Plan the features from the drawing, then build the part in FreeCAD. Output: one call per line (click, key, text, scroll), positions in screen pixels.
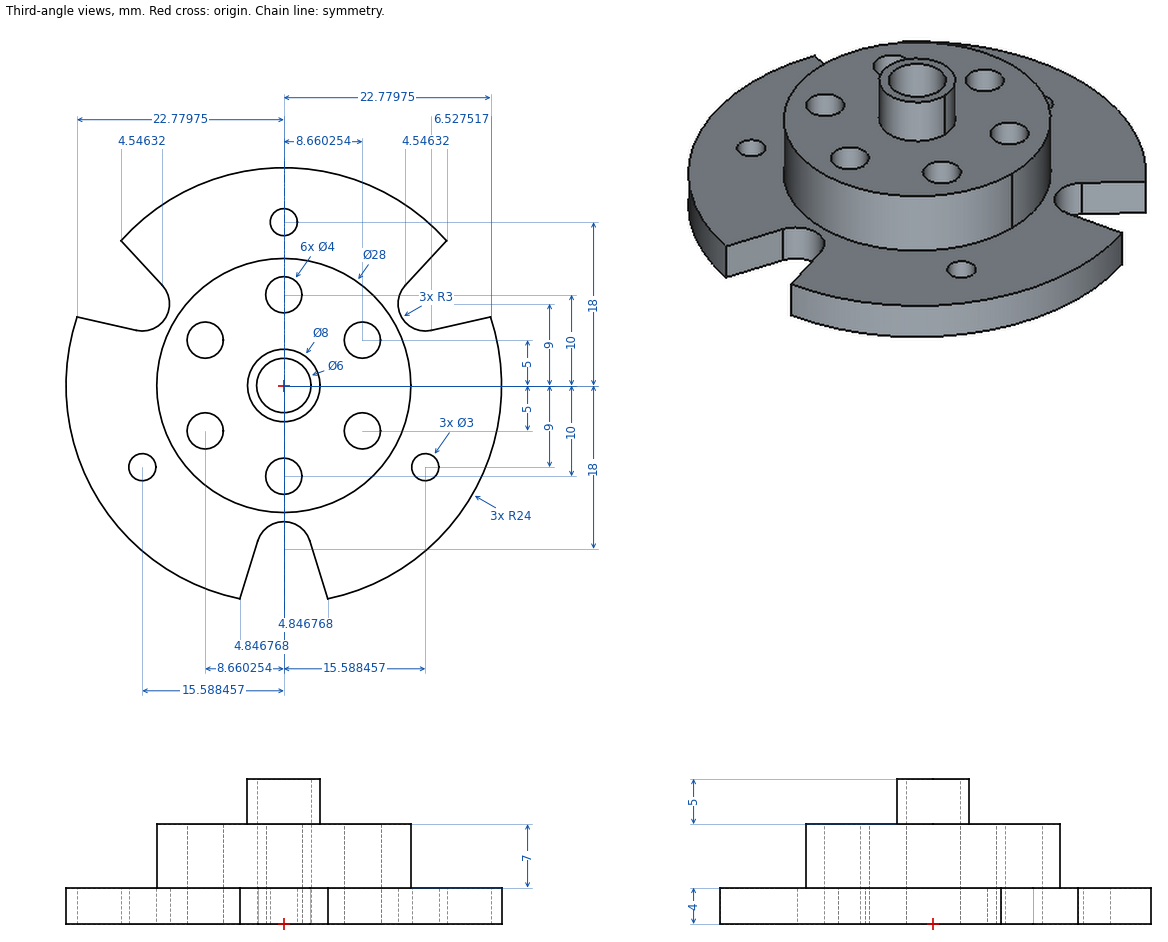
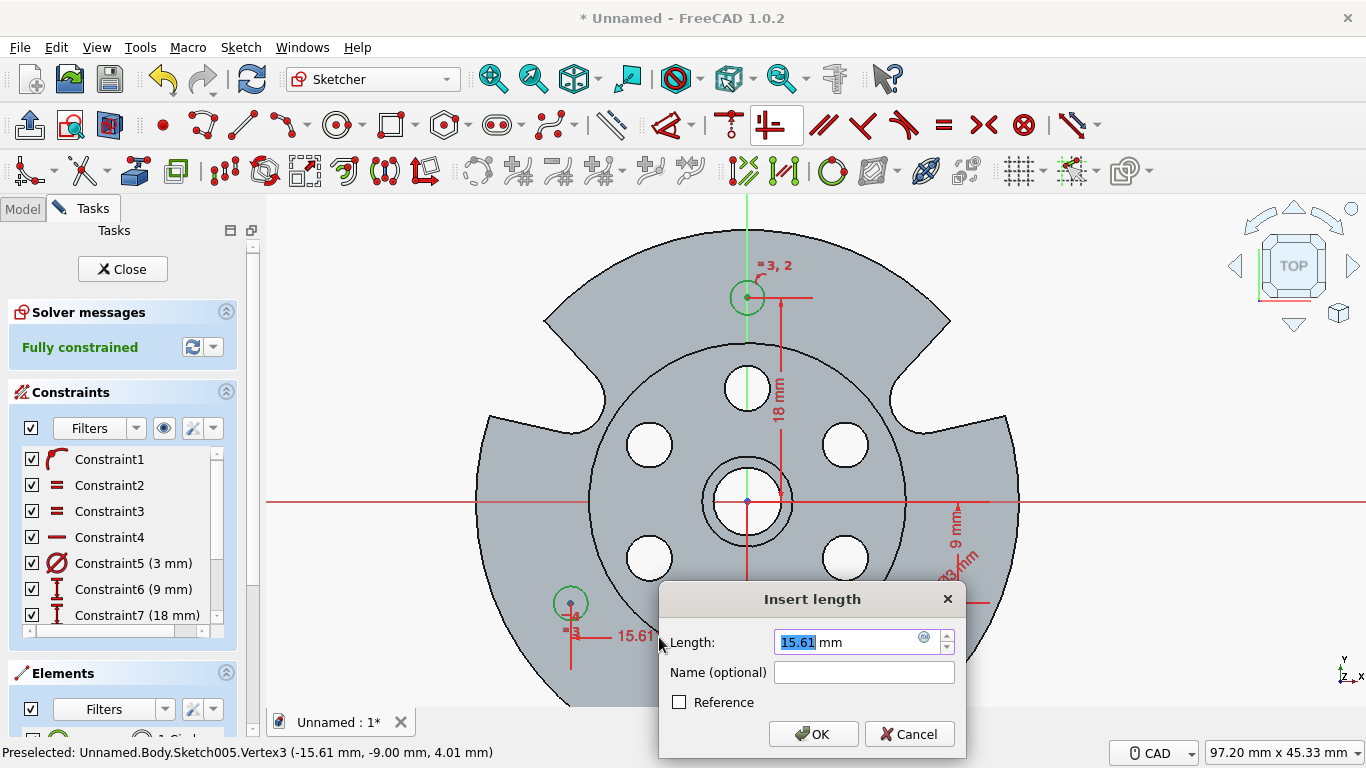
text(15.588457)
key(Return)
key(Escape)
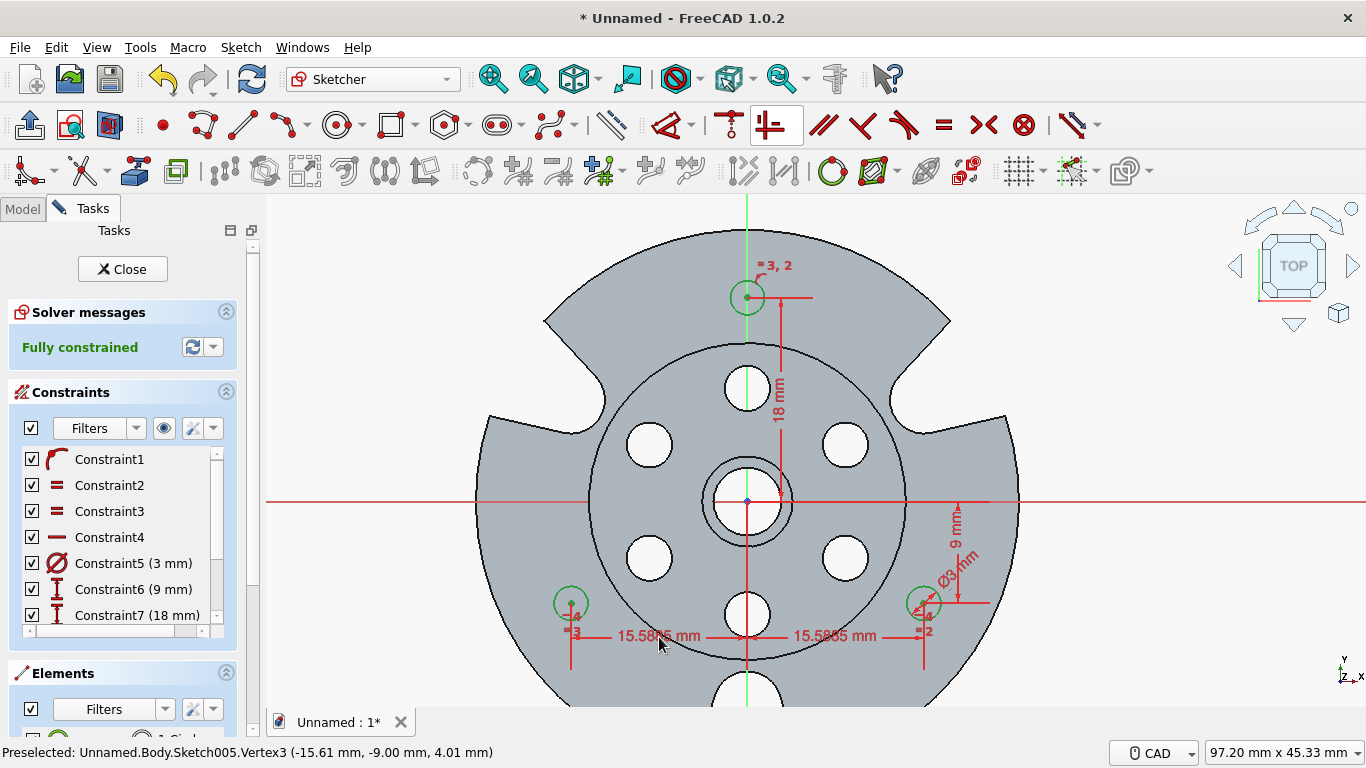
click(123, 269)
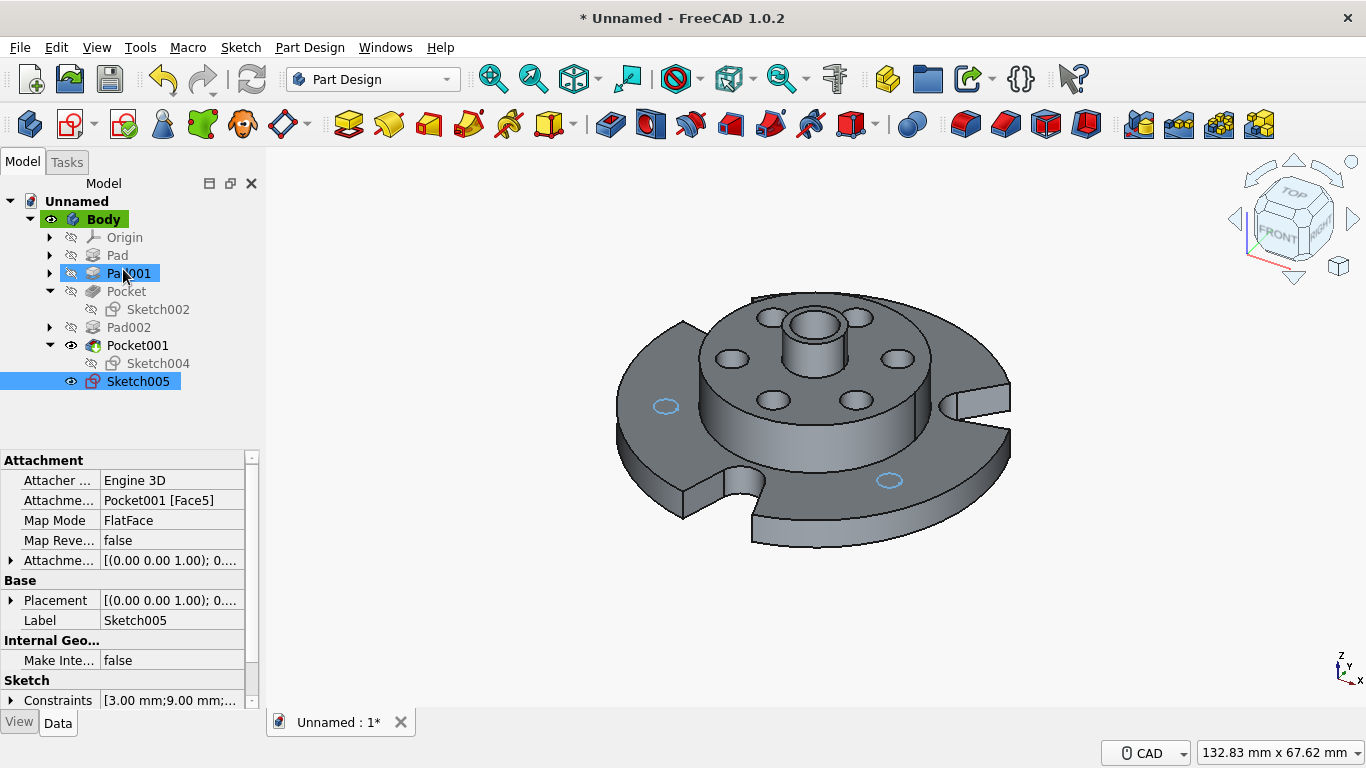
click(612, 124)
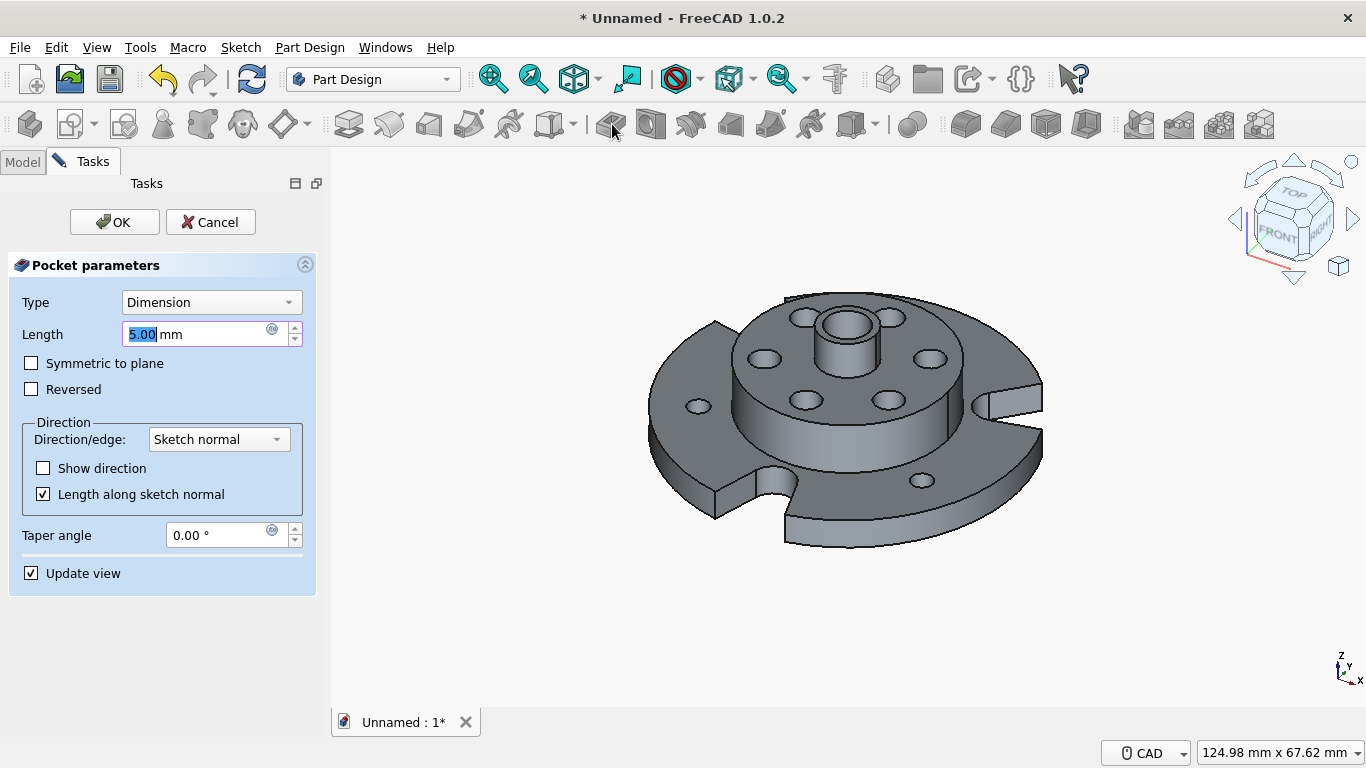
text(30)
key(Tab)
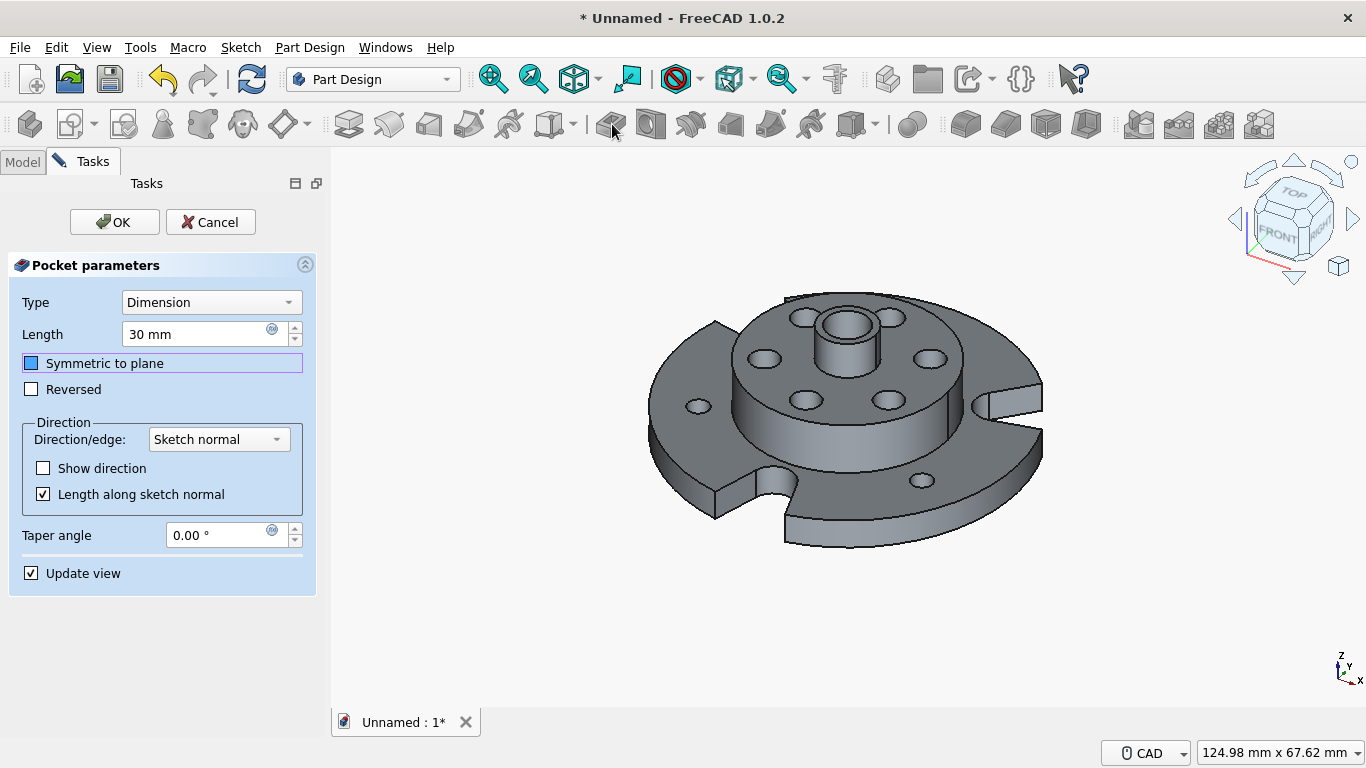
click(115, 222)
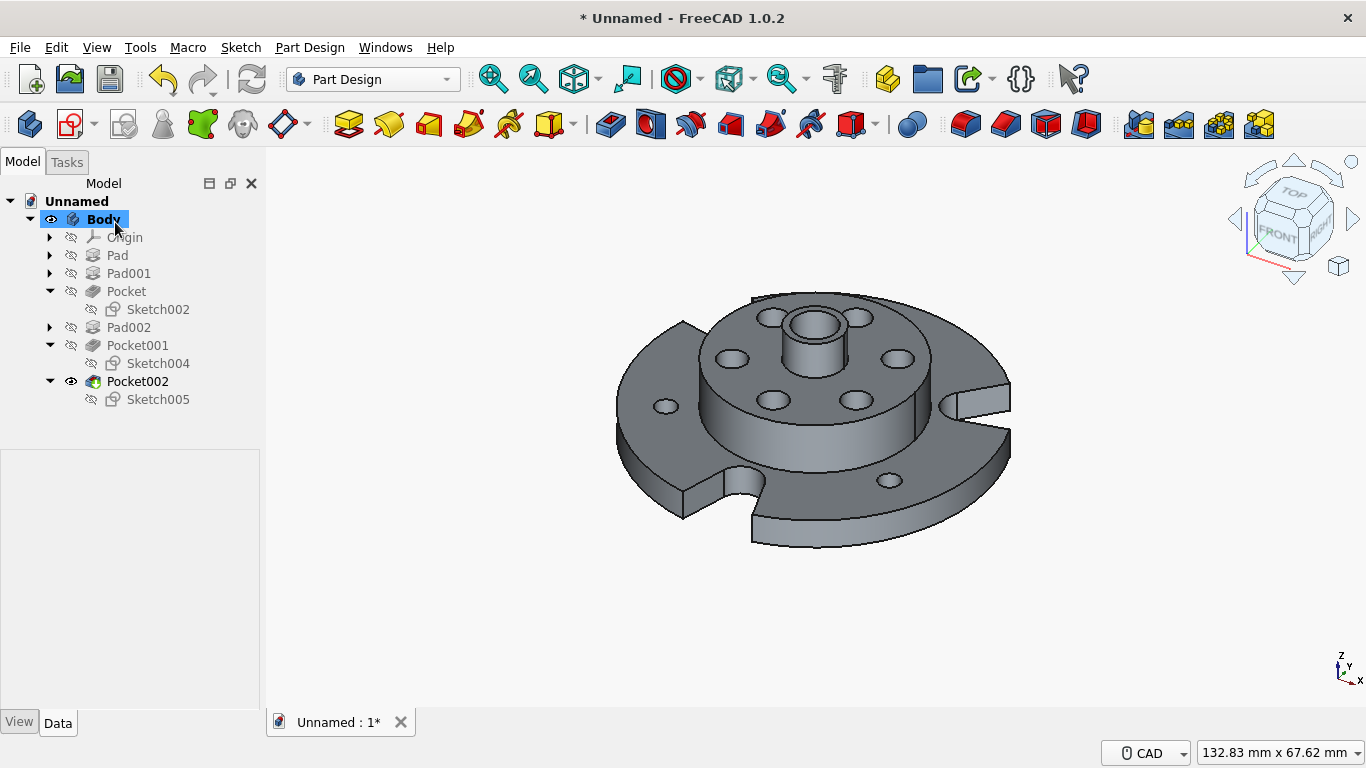
key(0)